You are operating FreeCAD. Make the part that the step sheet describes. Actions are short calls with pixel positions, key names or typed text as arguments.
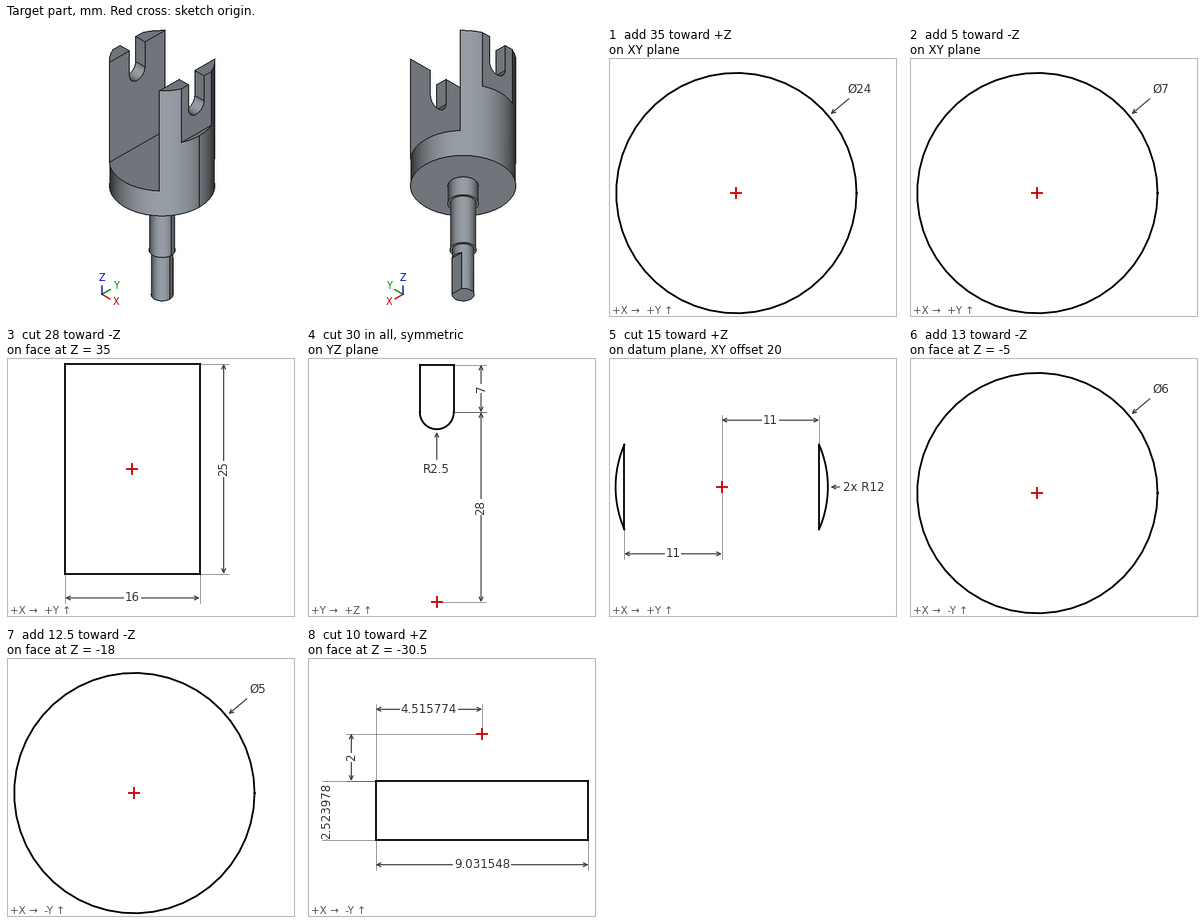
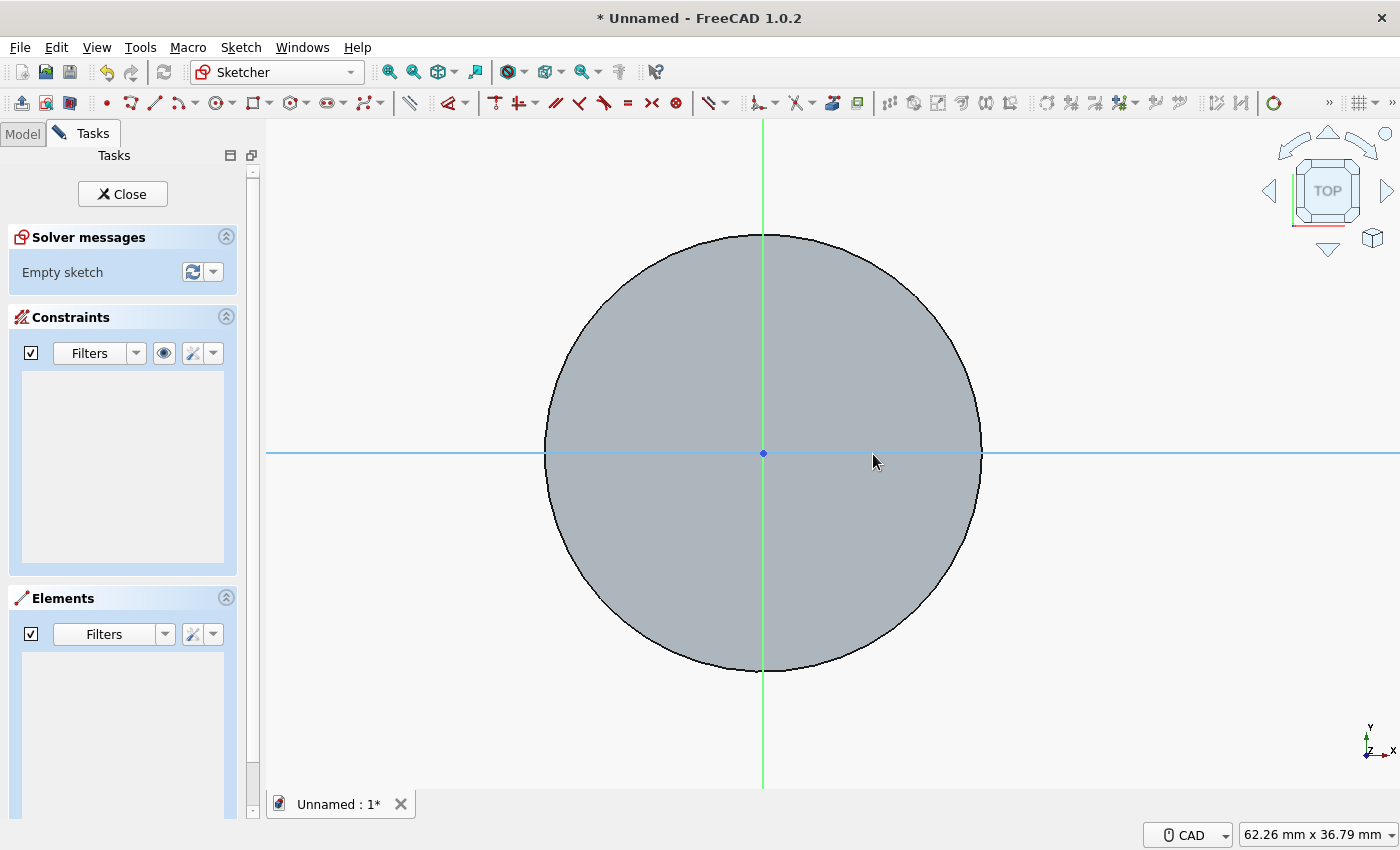
click(272, 104)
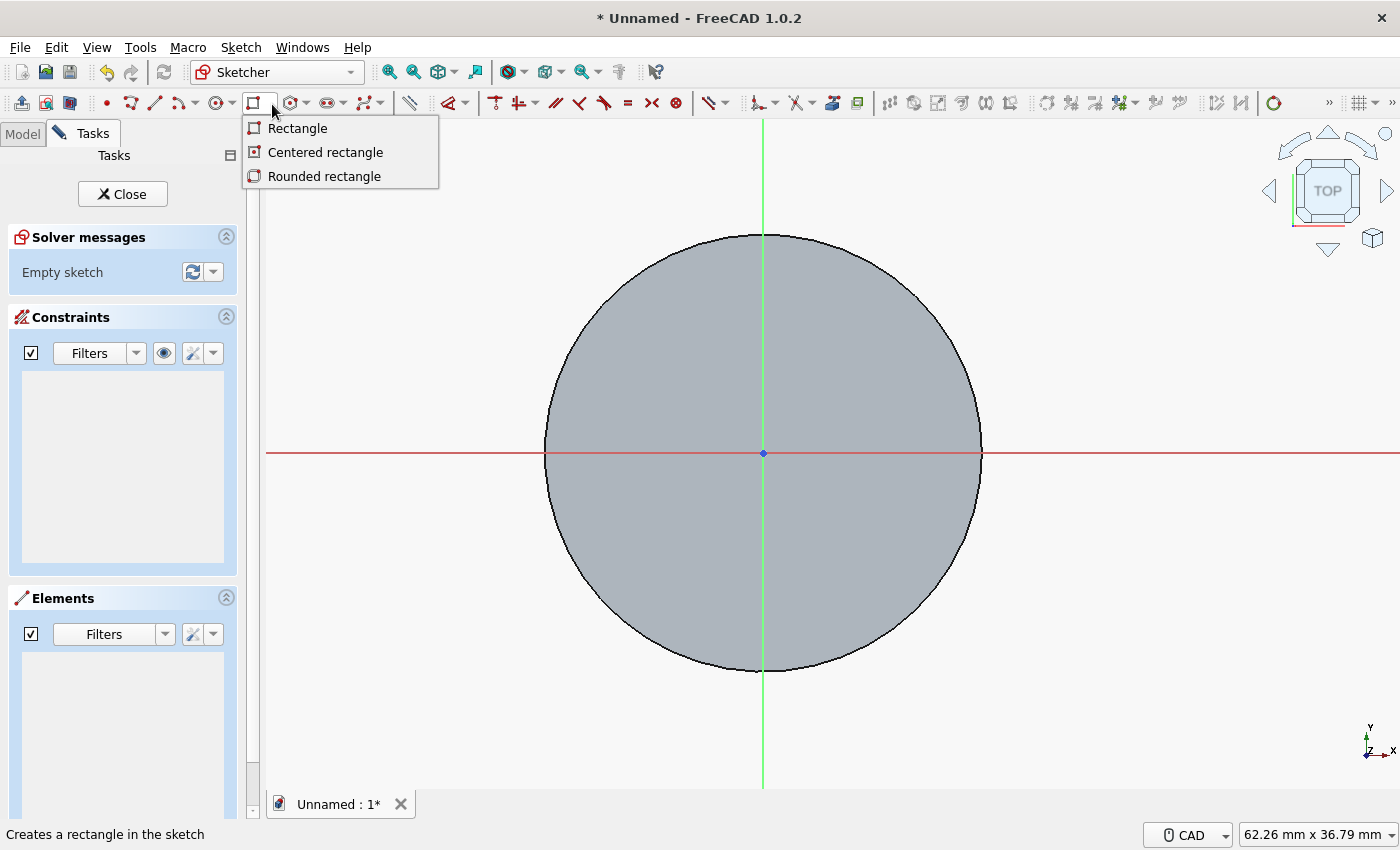
click(340, 152)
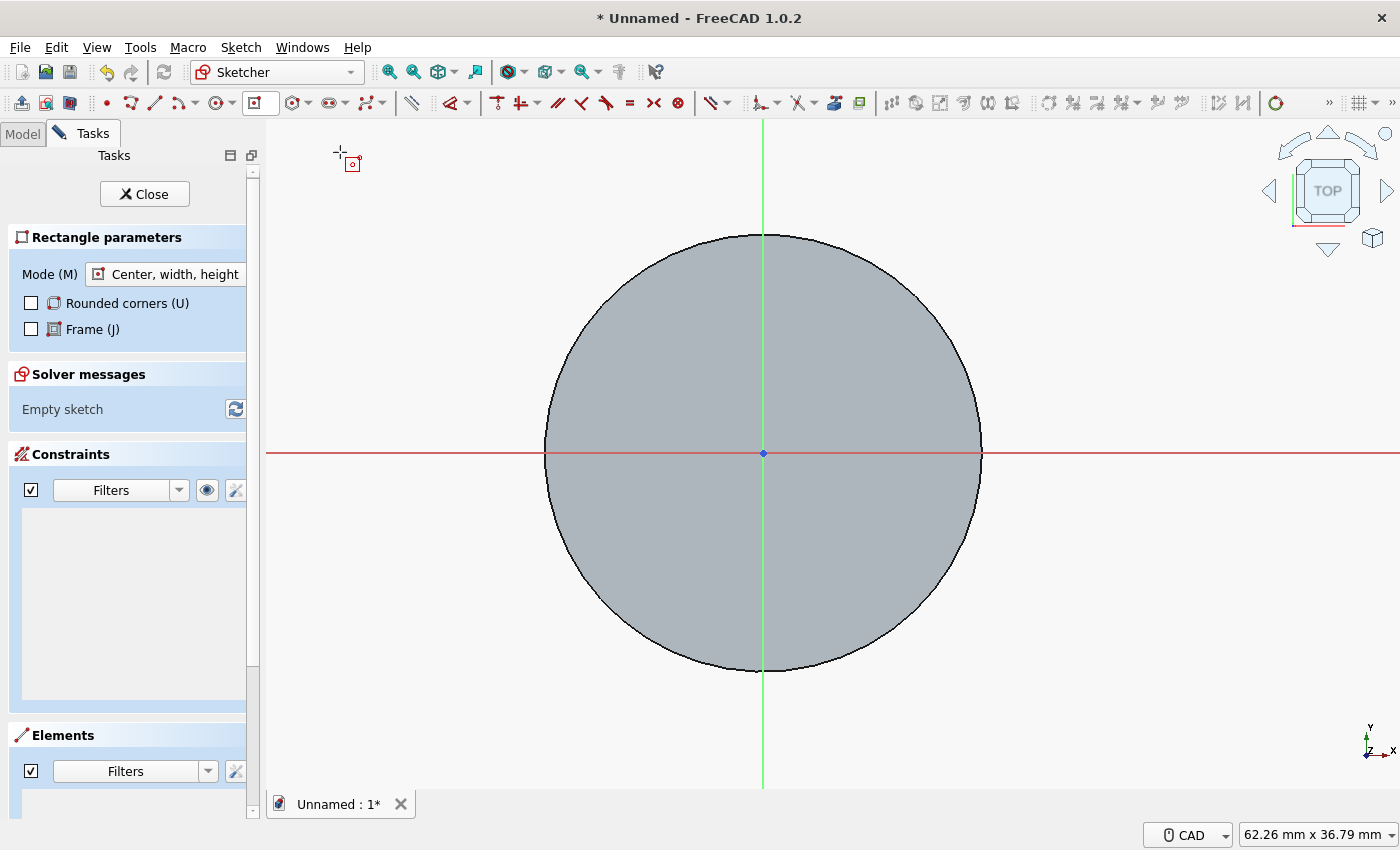
click(763, 453)
click(909, 225)
key(Escape)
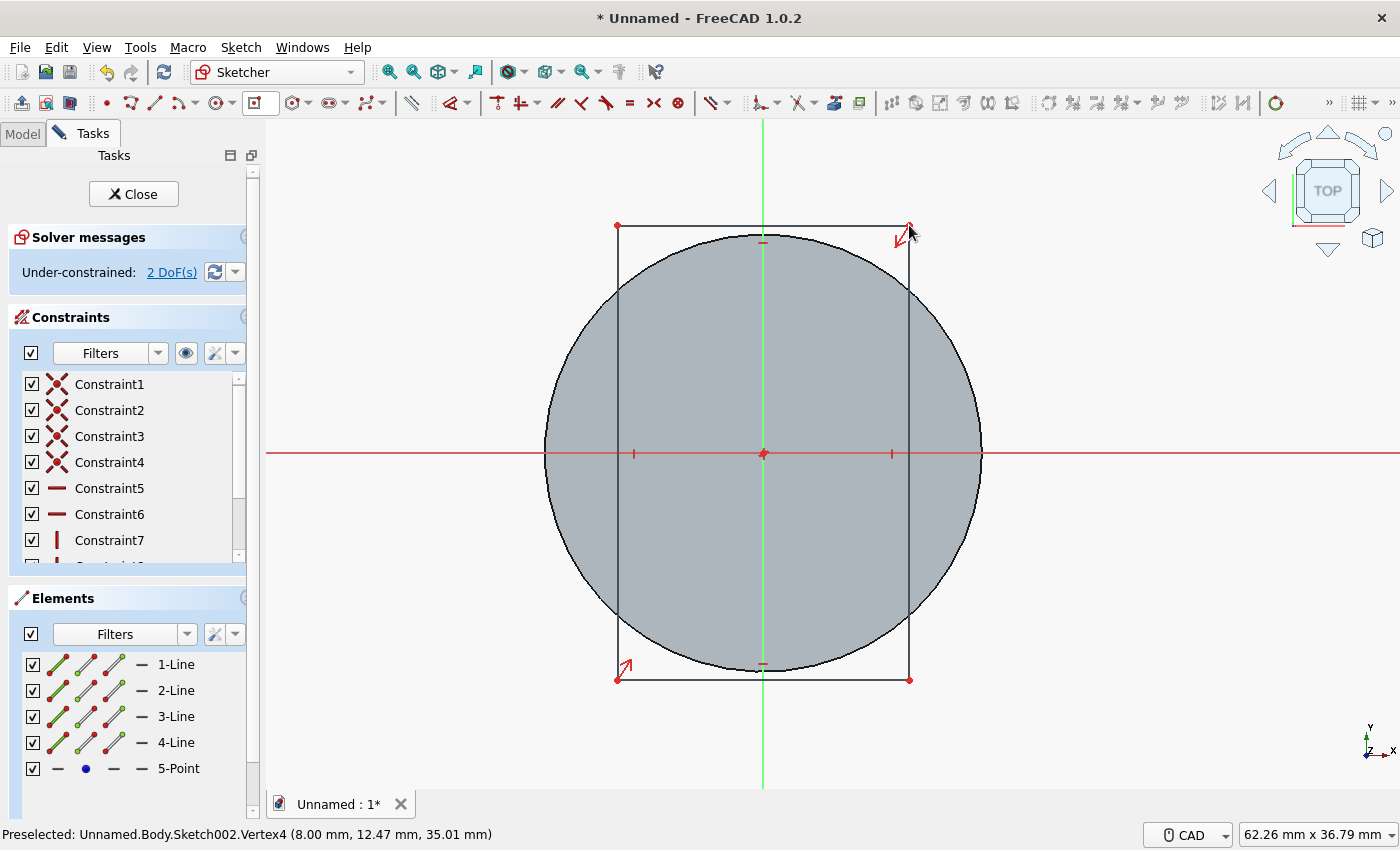
click(450, 104)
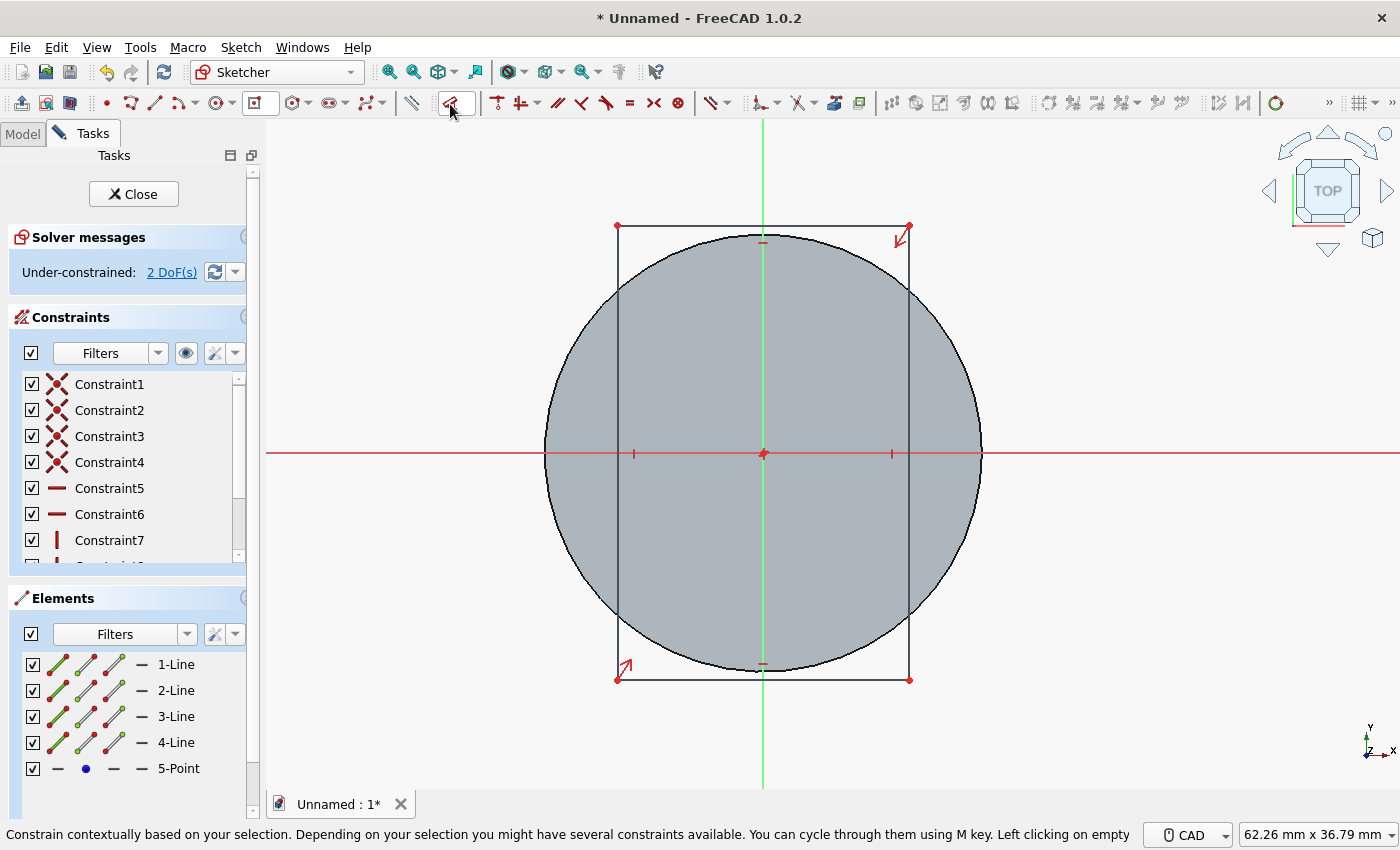
click(705, 680)
click(696, 714)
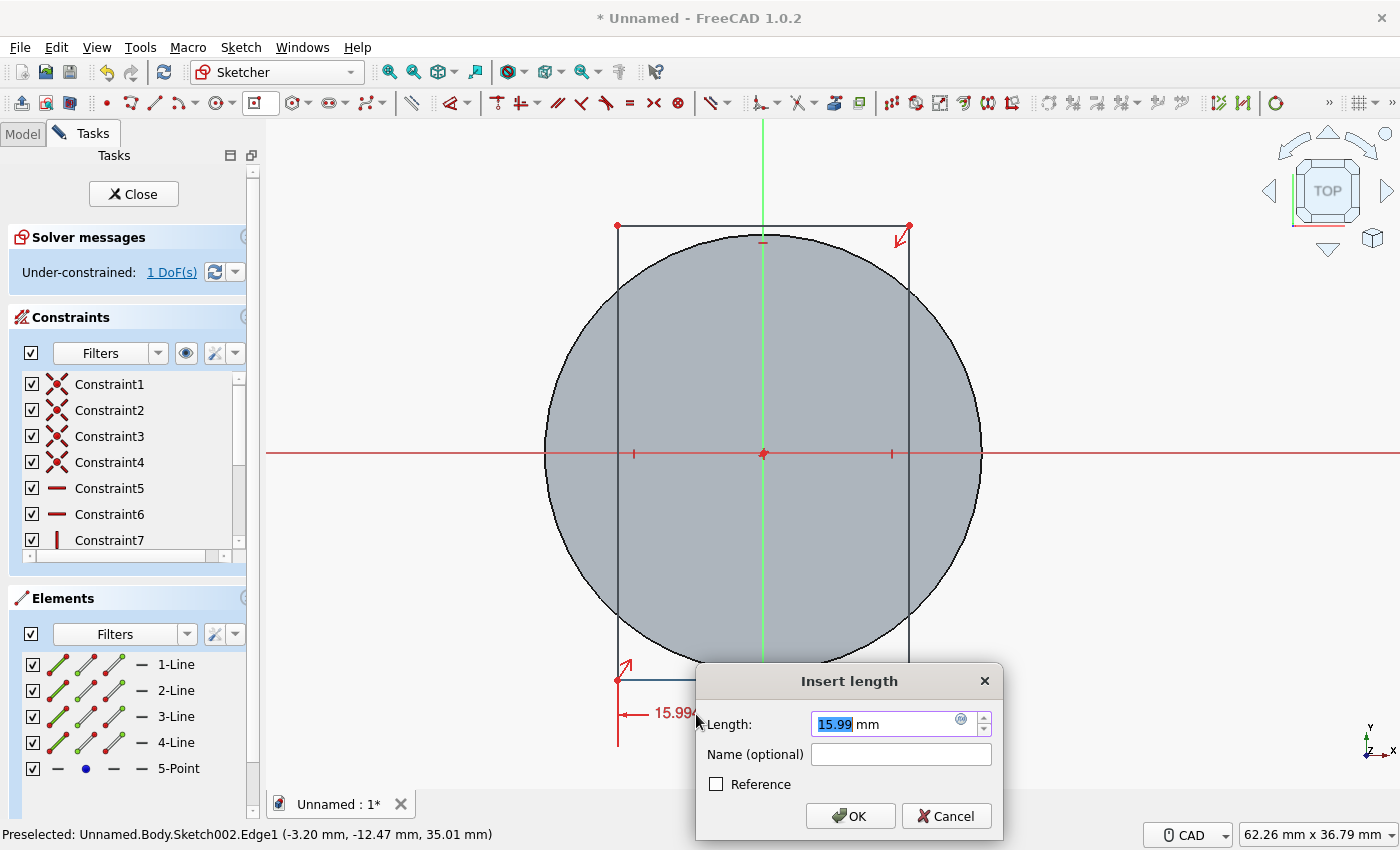
text(16)
key(Return)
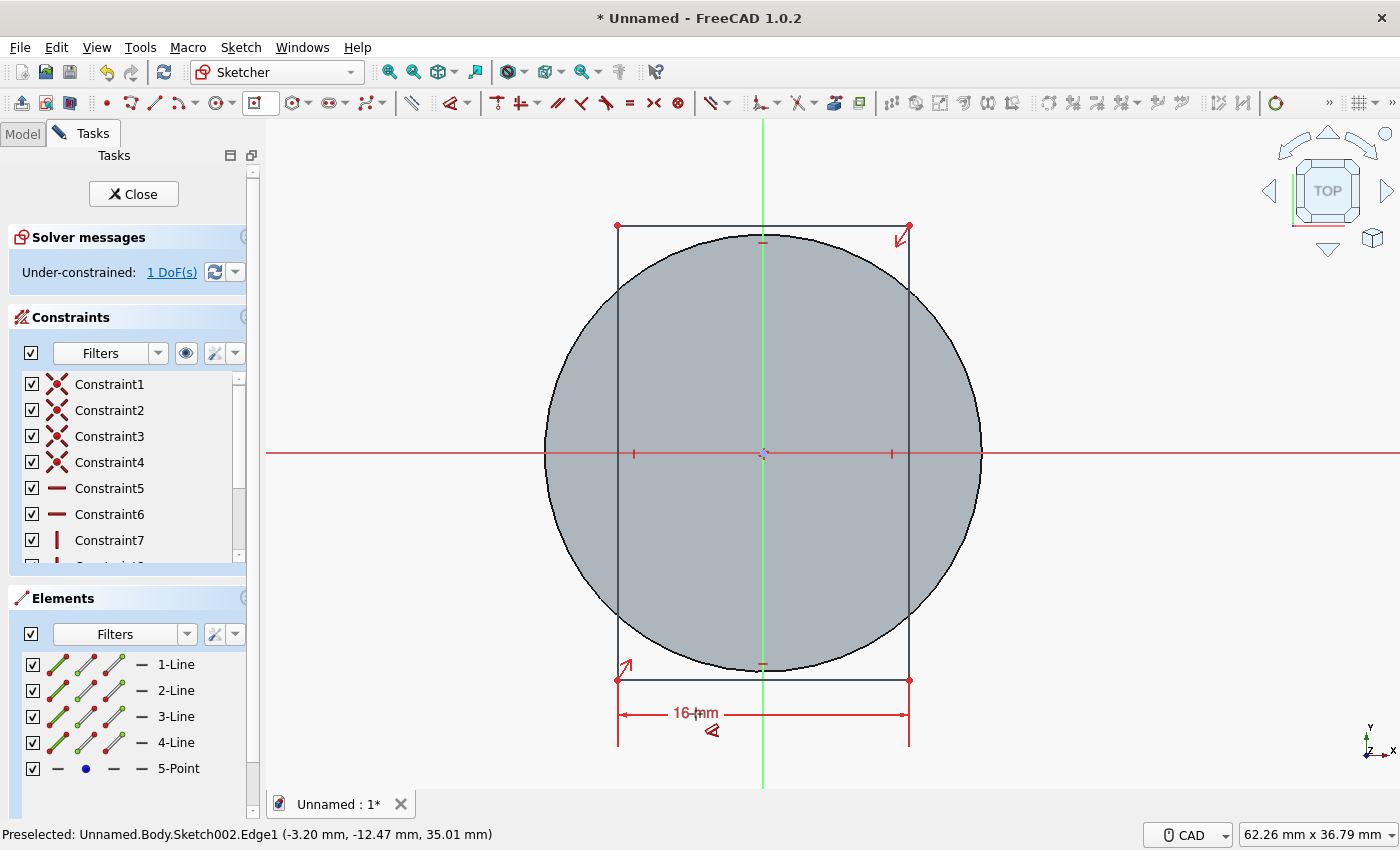
click(909, 544)
click(943, 349)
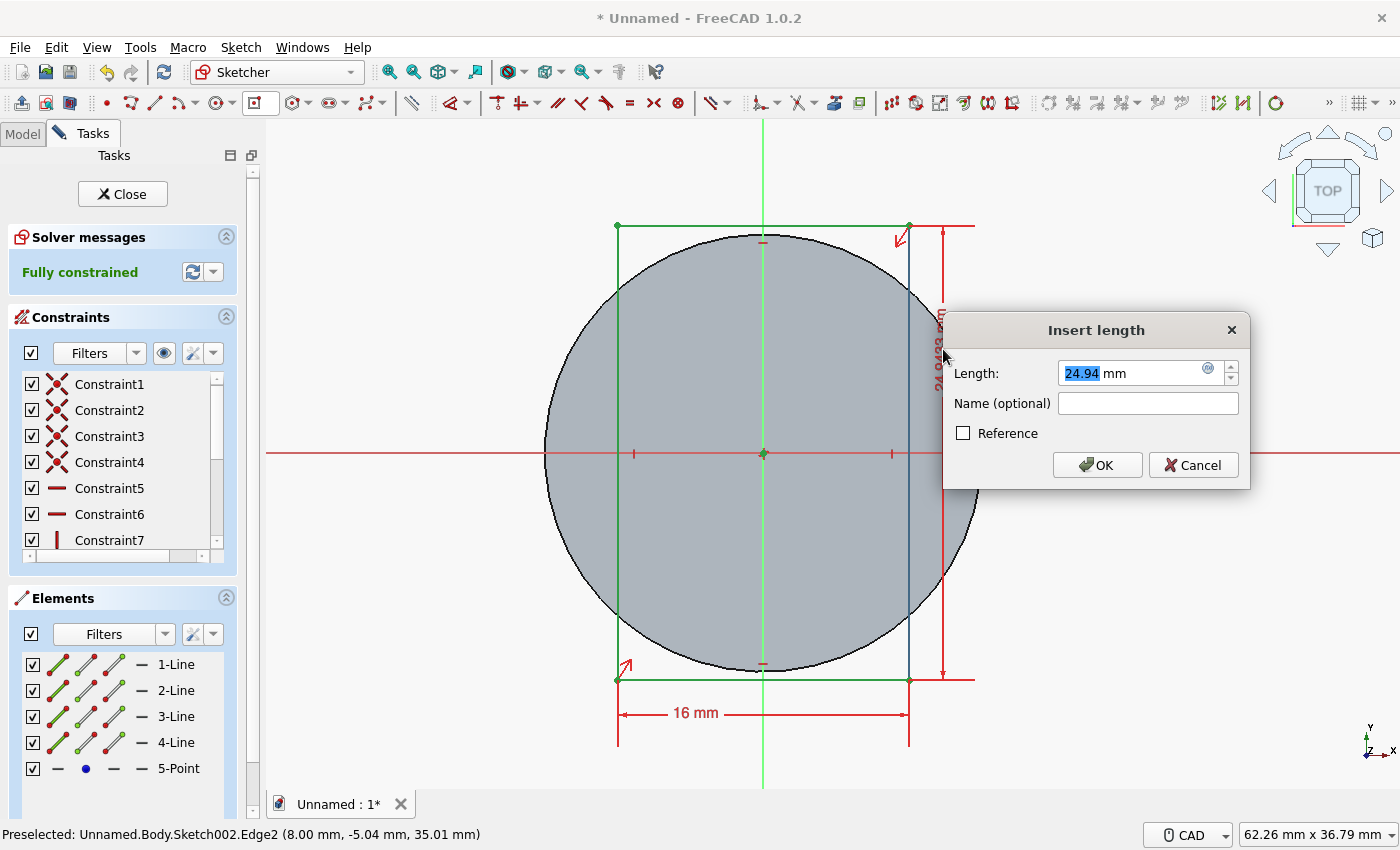
text(25)
key(Return)
key(Escape)